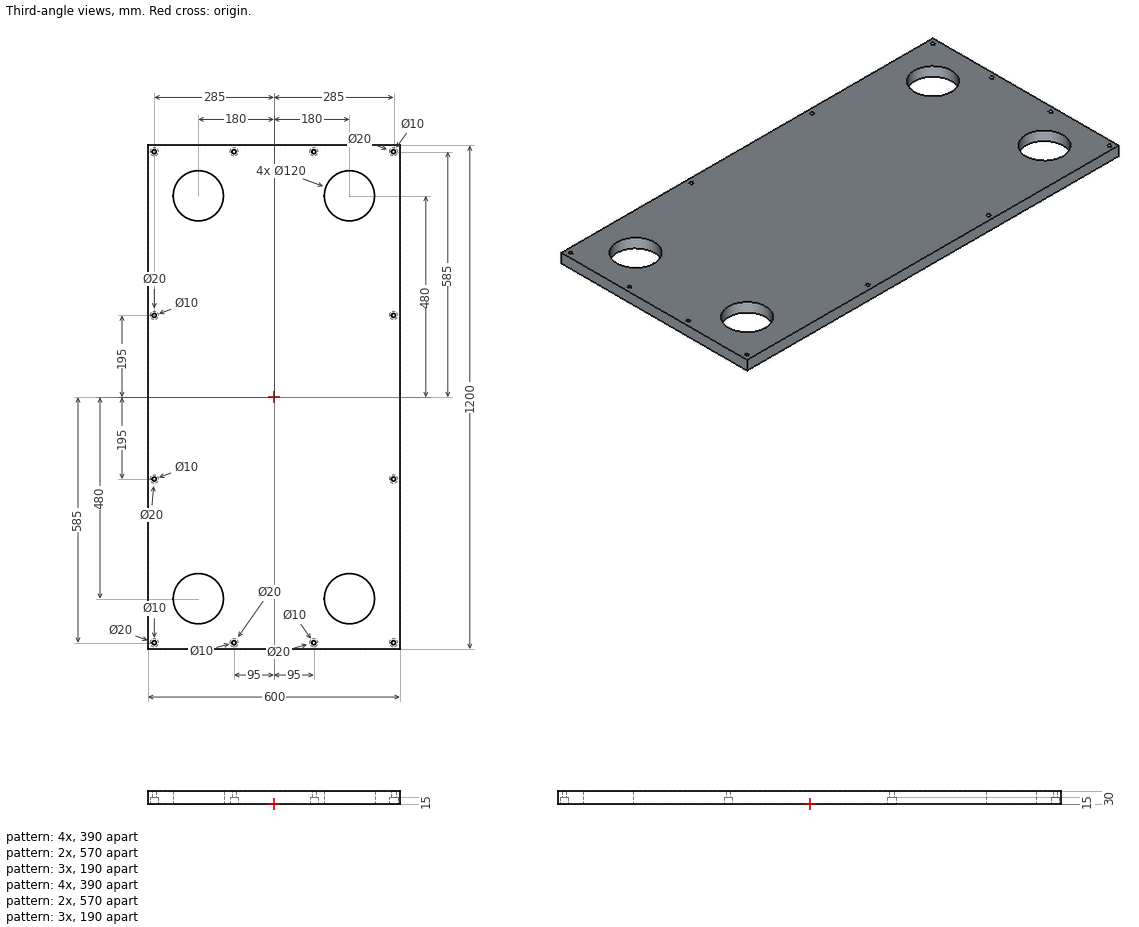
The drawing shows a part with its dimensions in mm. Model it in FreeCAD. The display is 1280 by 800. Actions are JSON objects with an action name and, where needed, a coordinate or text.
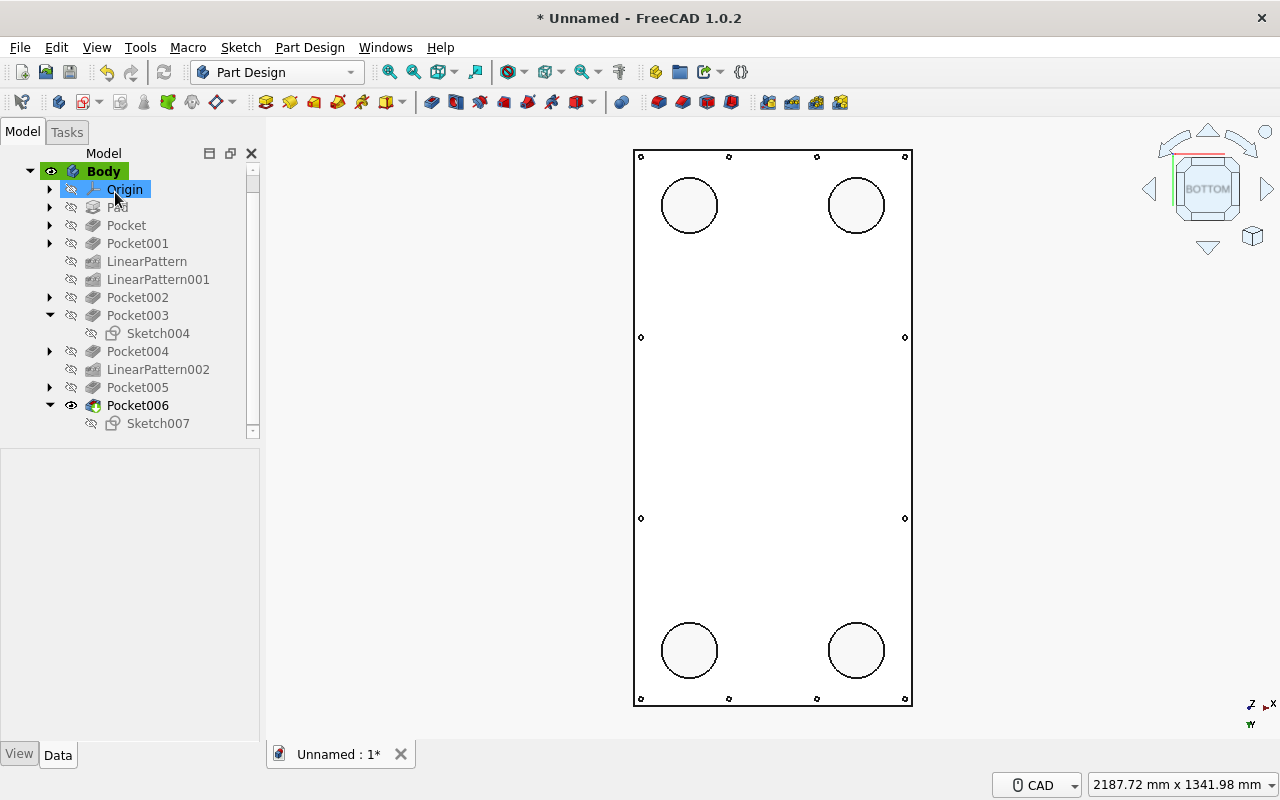
{"action": "left_click", "coordinate": [84, 102]}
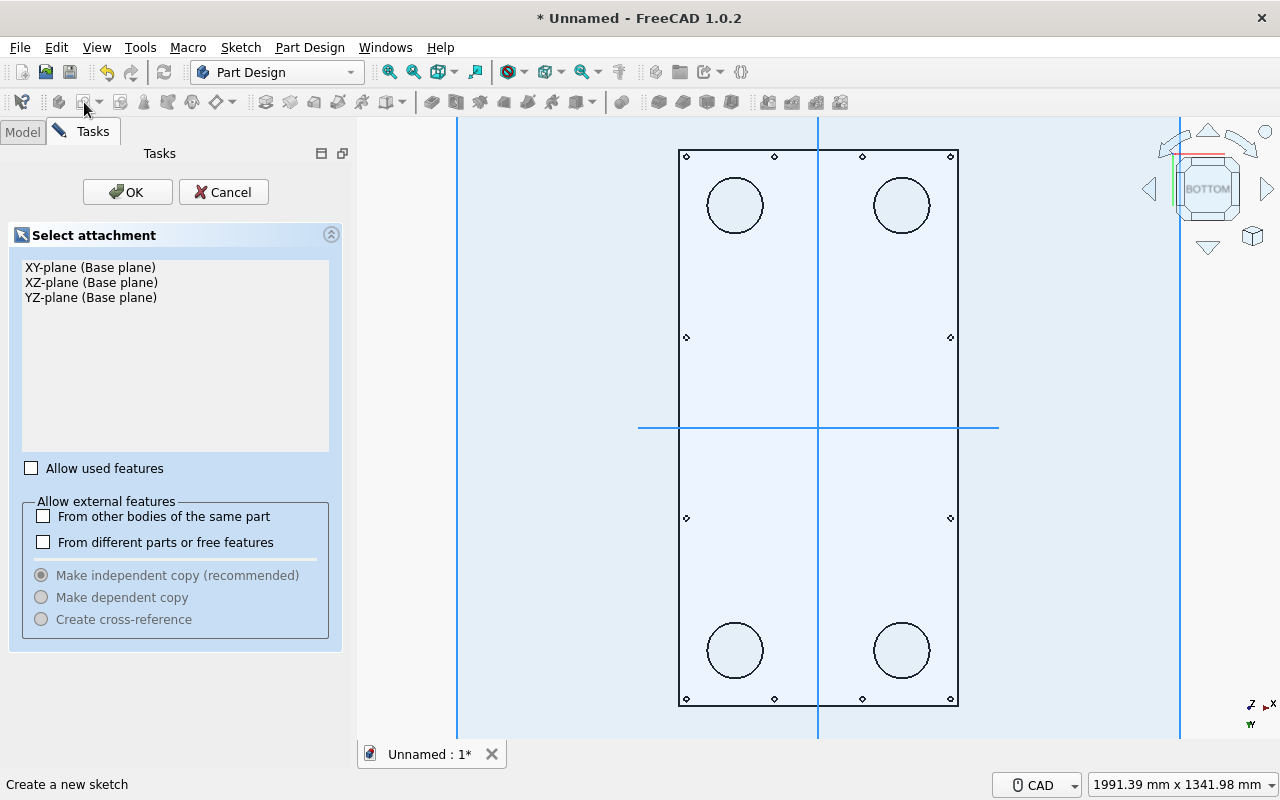
{"action": "left_click", "coordinate": [82, 268]}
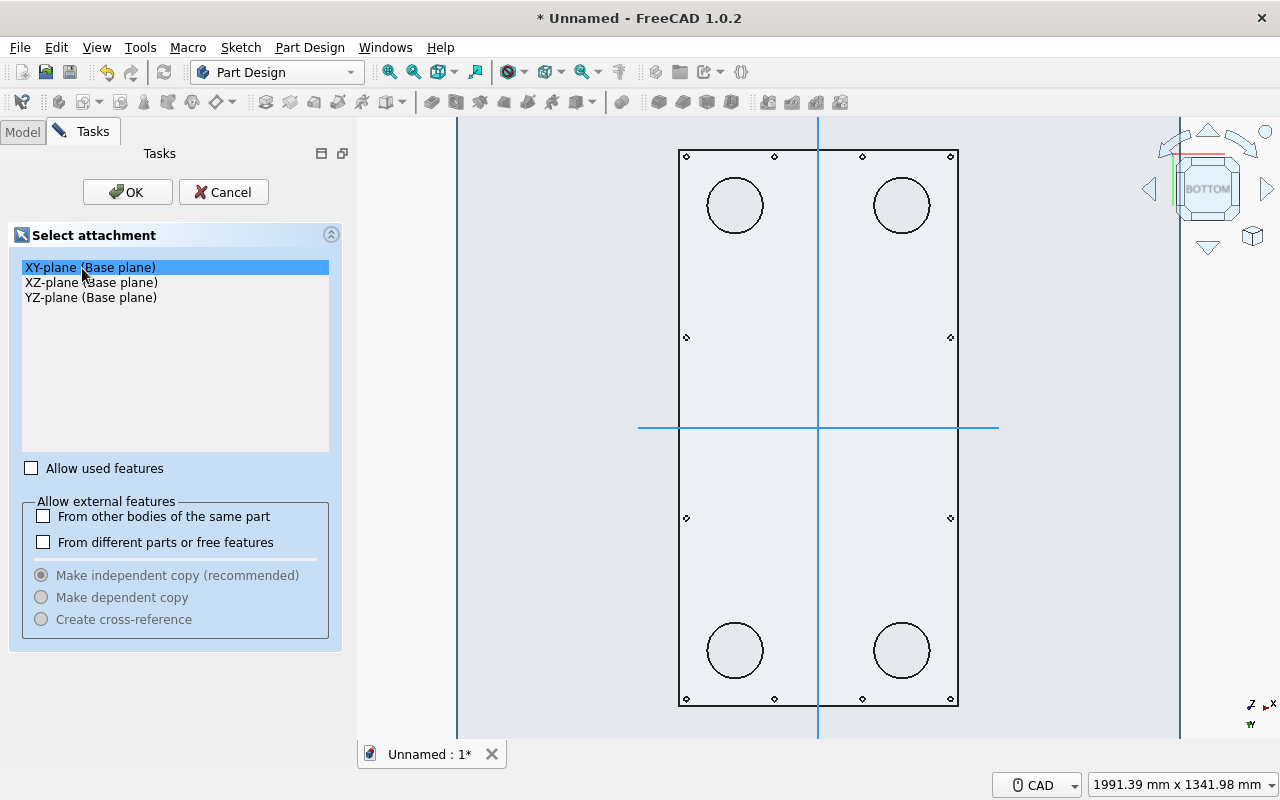
{"action": "left_click", "coordinate": [128, 192]}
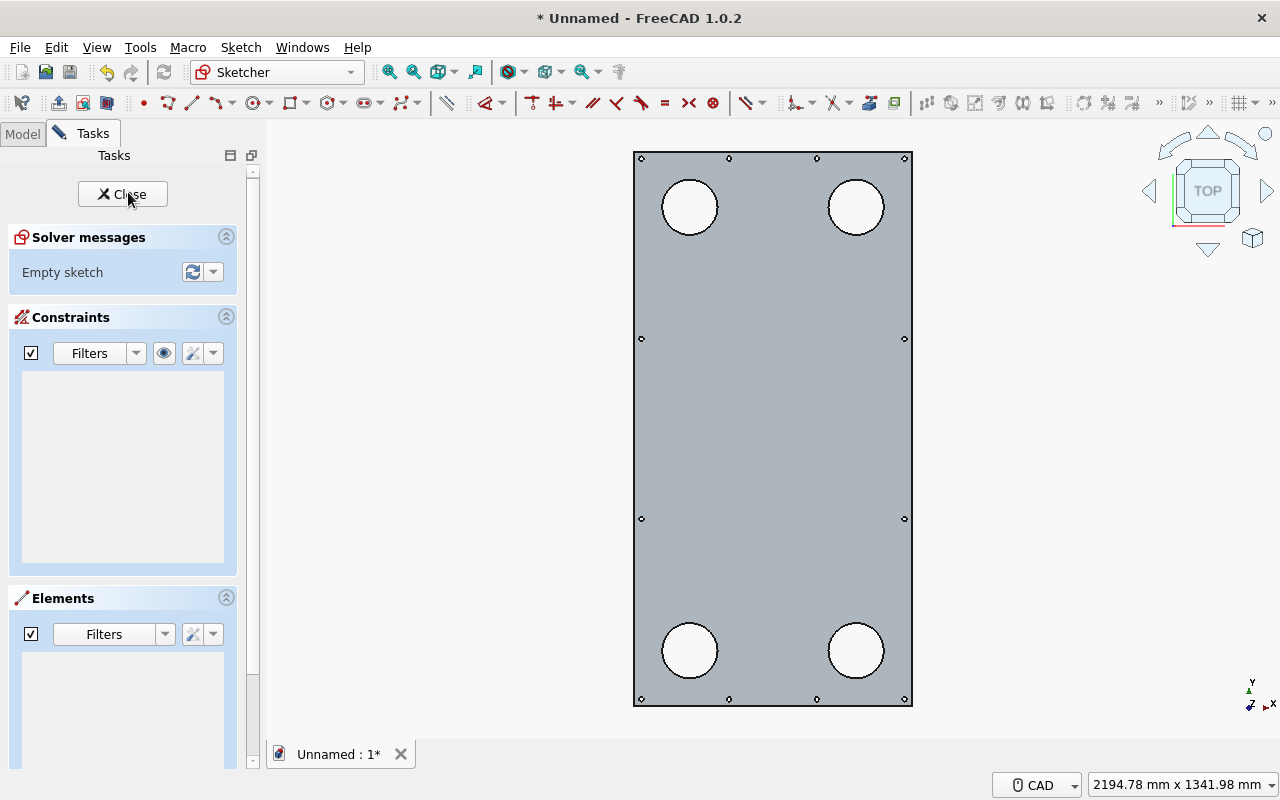
{"action": "left_click", "coordinate": [108, 104]}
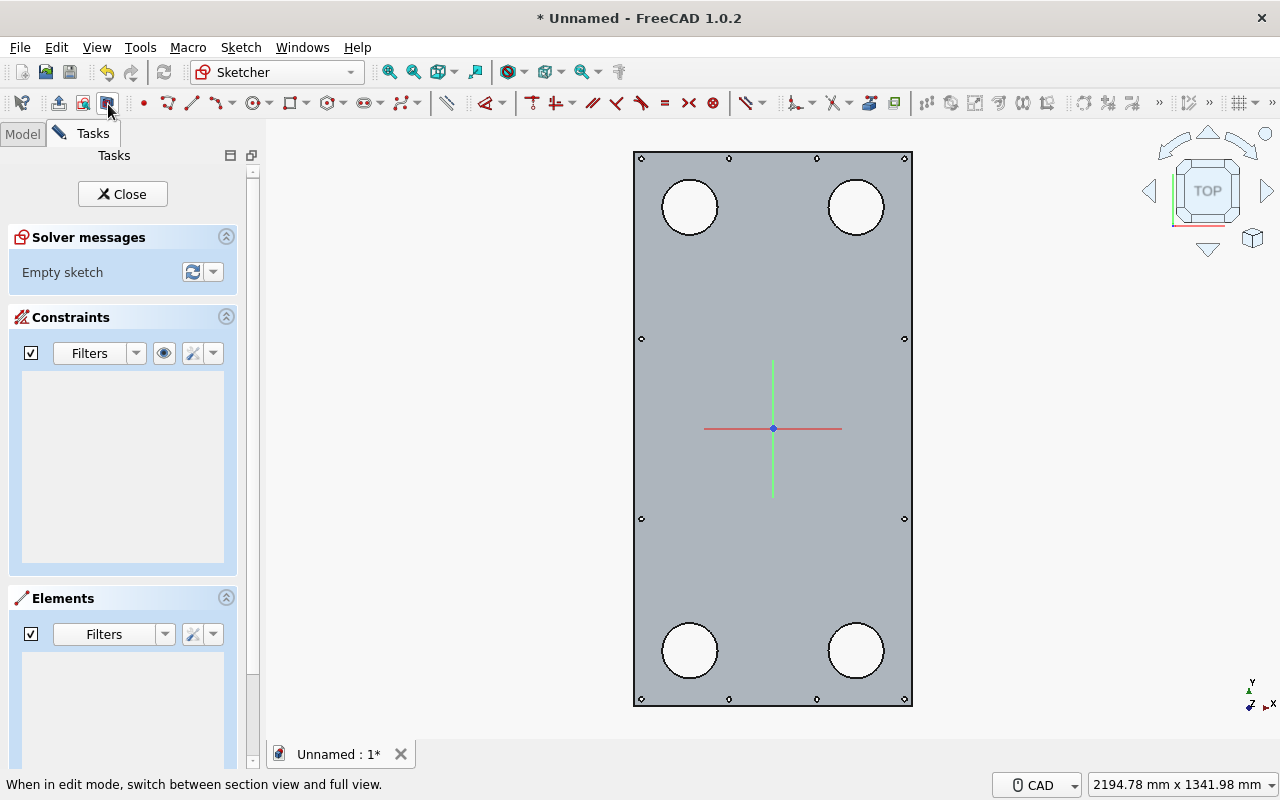
{"action": "scroll", "coordinate": [915, 147], "scroll_direction": "up", "scroll_amount": 15}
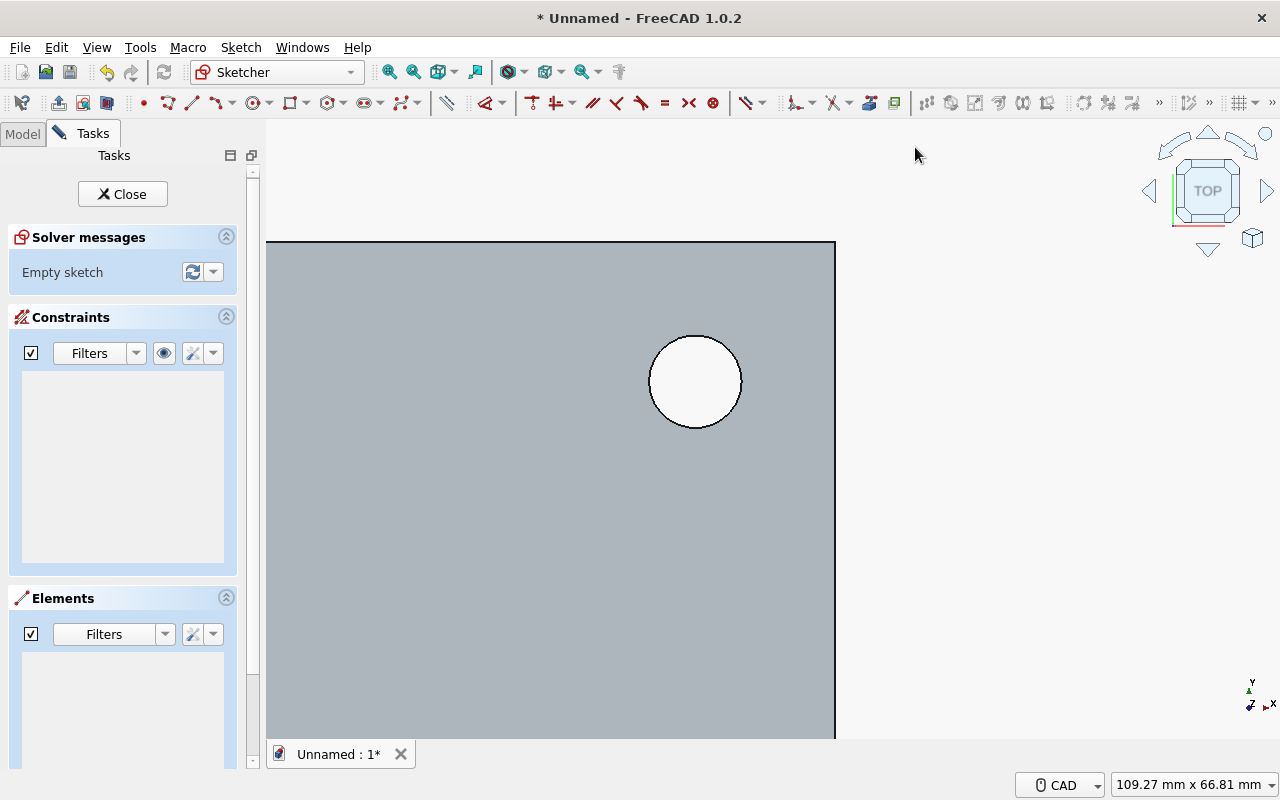
{"action": "scroll", "coordinate": [688, 343], "scroll_direction": "up", "scroll_amount": 4}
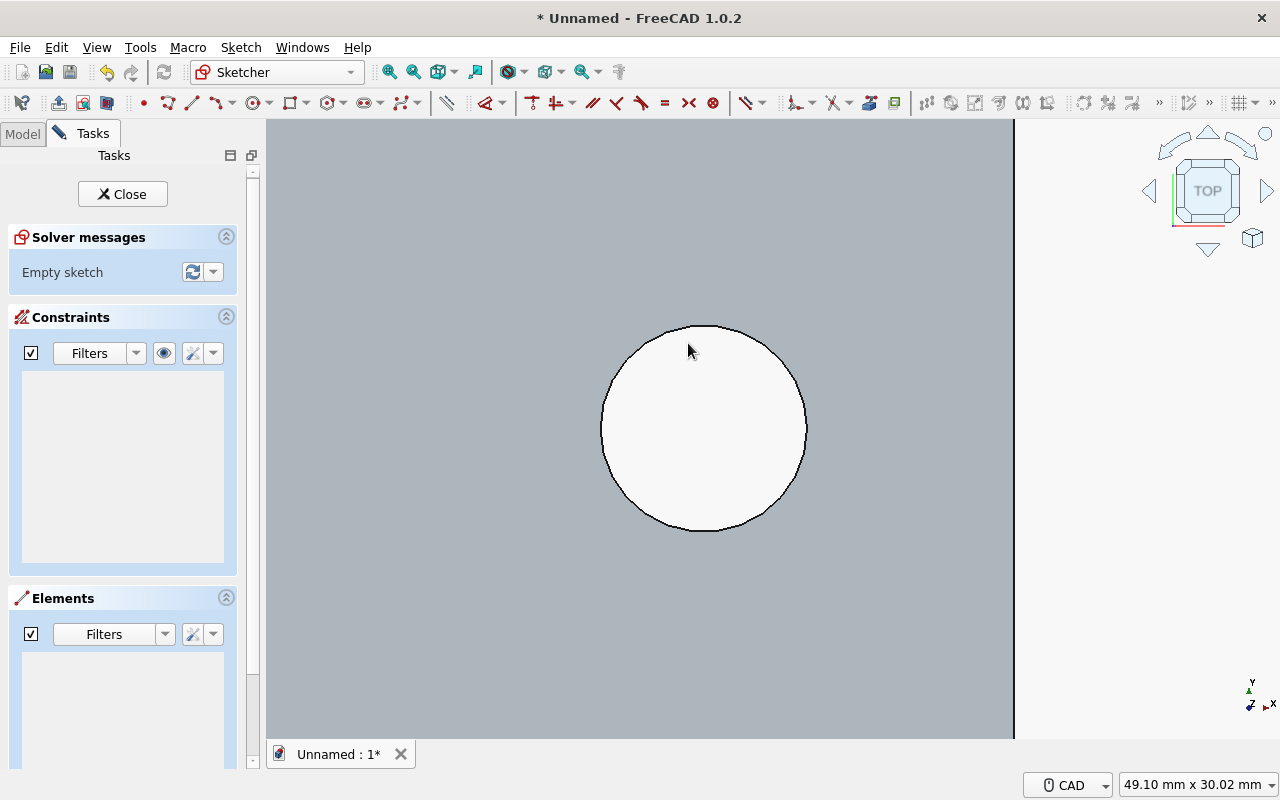
{"action": "left_click", "coordinate": [254, 104]}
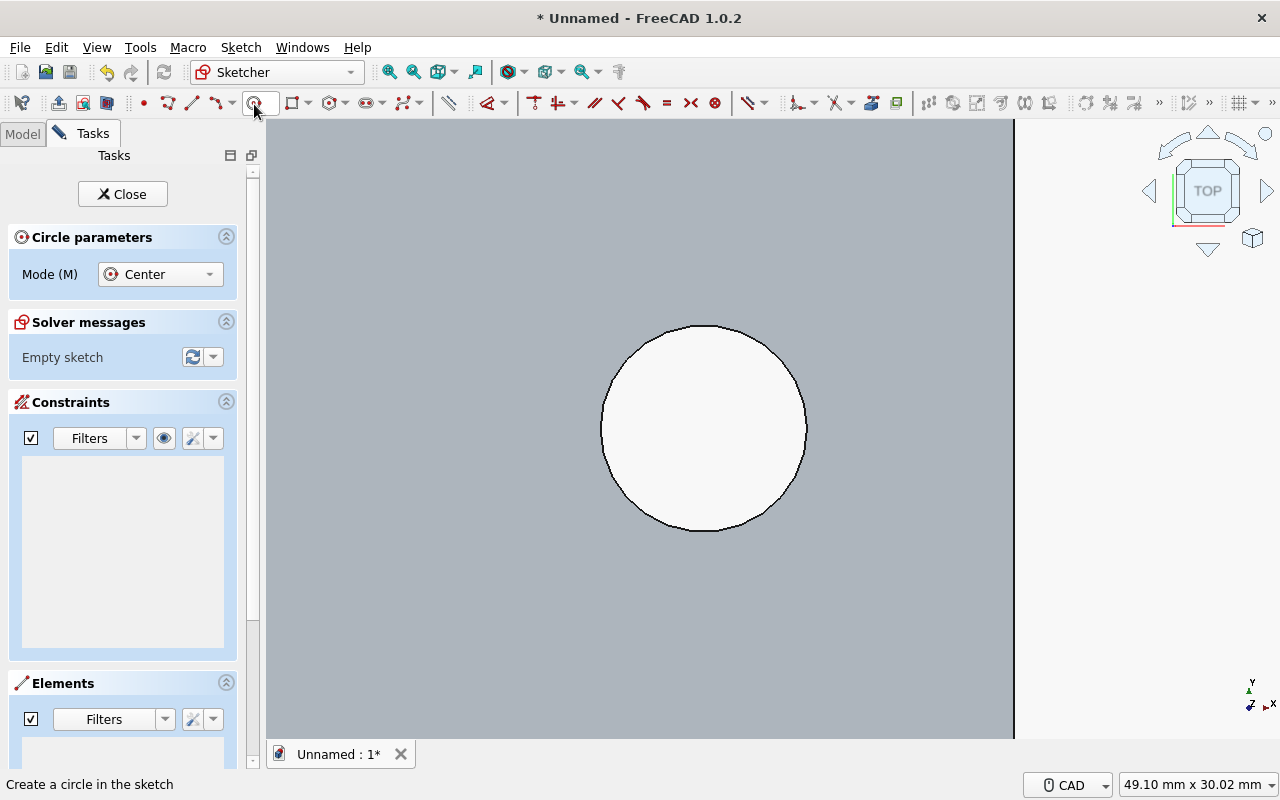
{"action": "left_click", "coordinate": [704, 429]}
{"action": "mouse_move", "coordinate": [850, 283]}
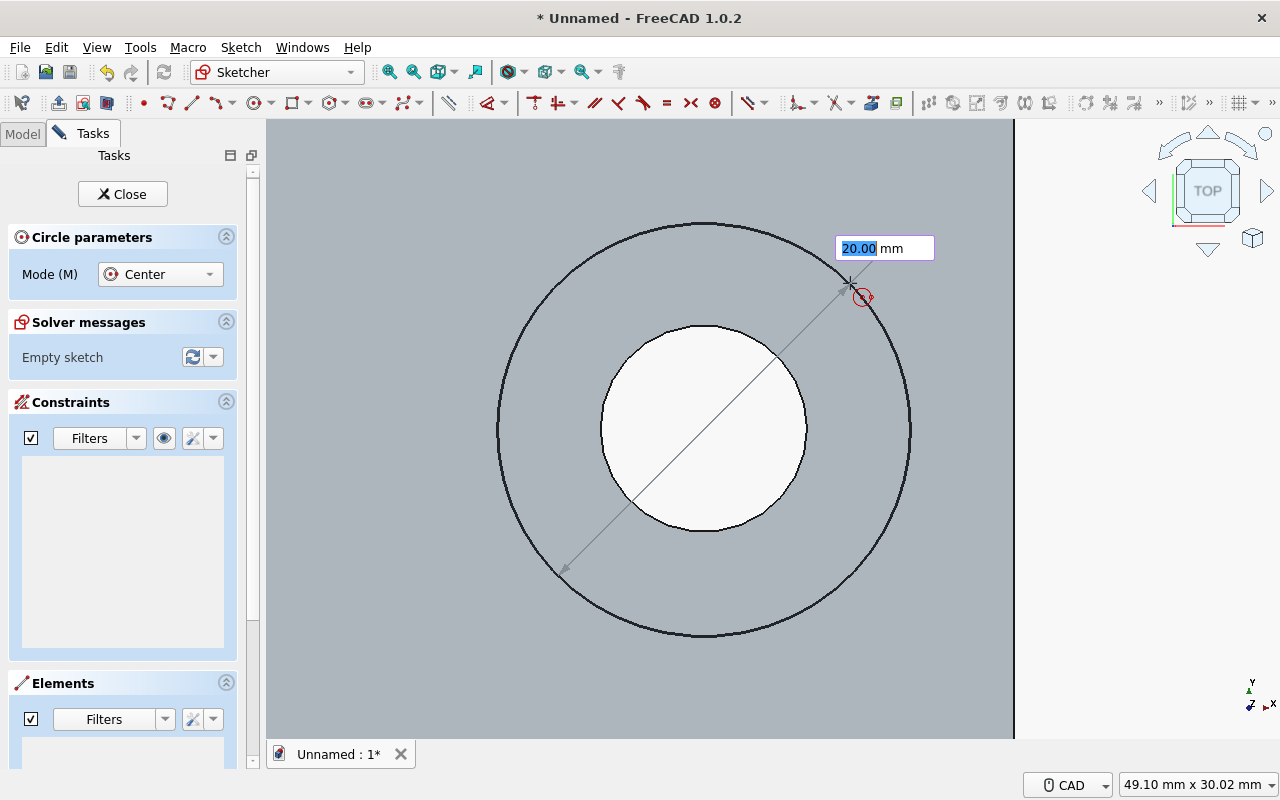
{"action": "type", "text": "20"}
{"action": "key", "text": "Return"}
{"action": "key", "text": "Escape"}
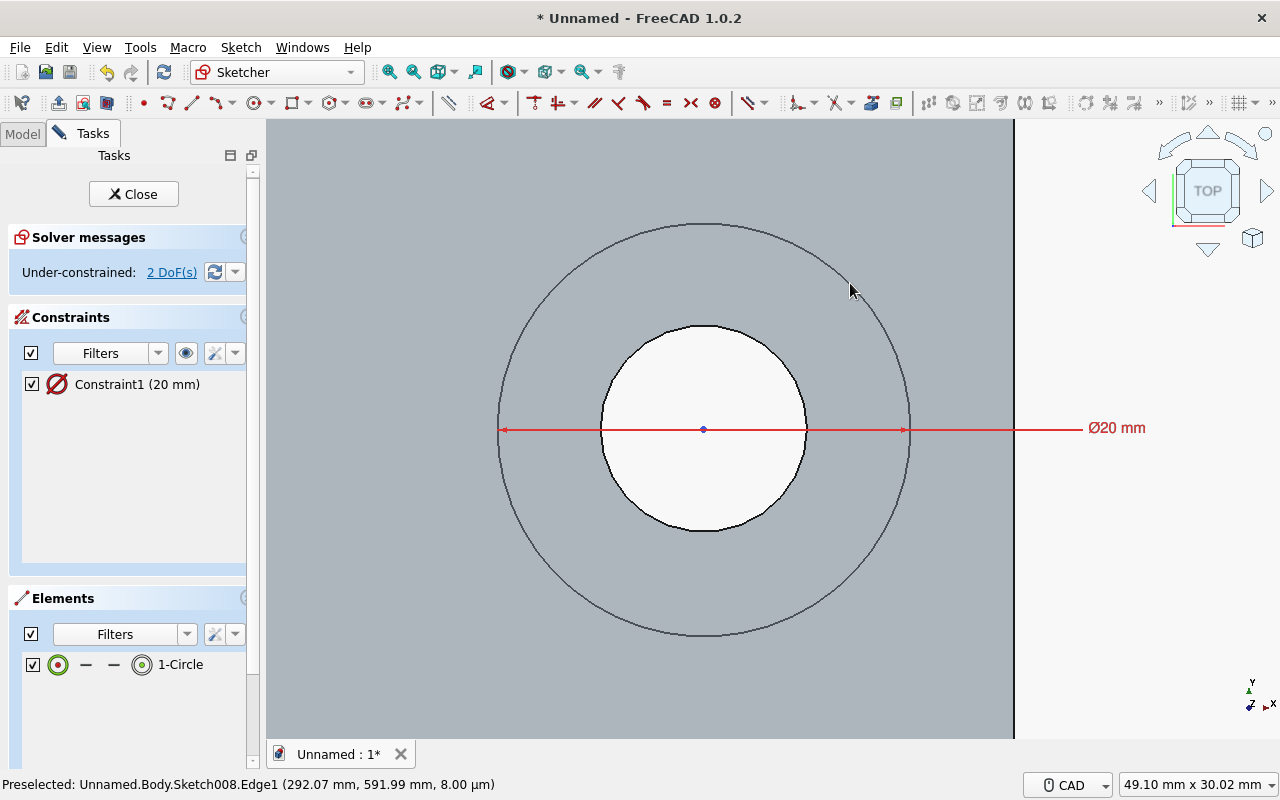
{"action": "left_click", "coordinate": [488, 104]}